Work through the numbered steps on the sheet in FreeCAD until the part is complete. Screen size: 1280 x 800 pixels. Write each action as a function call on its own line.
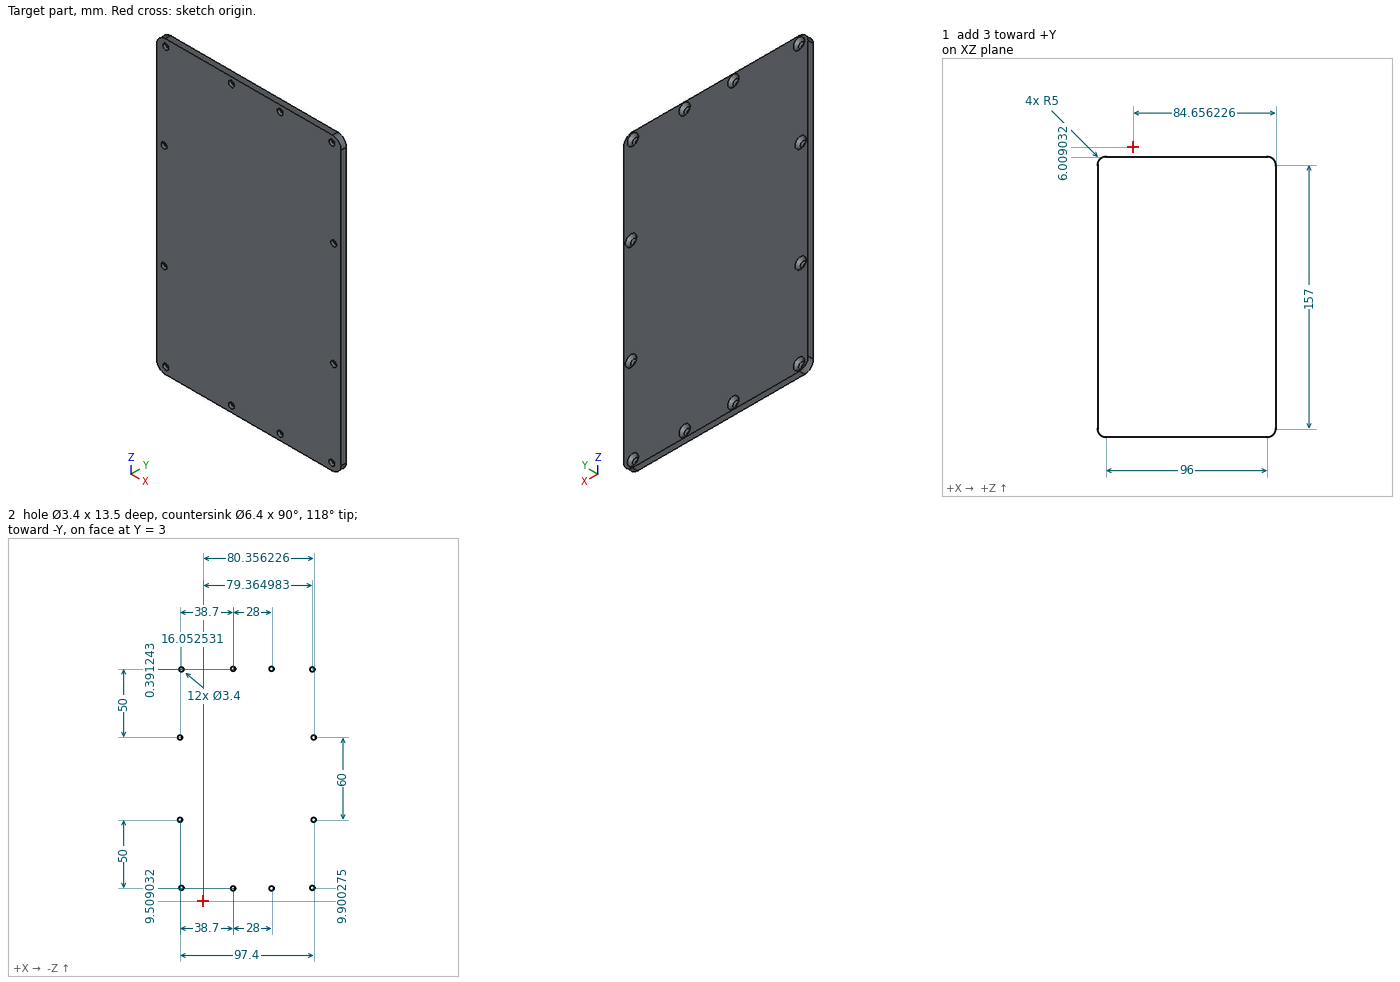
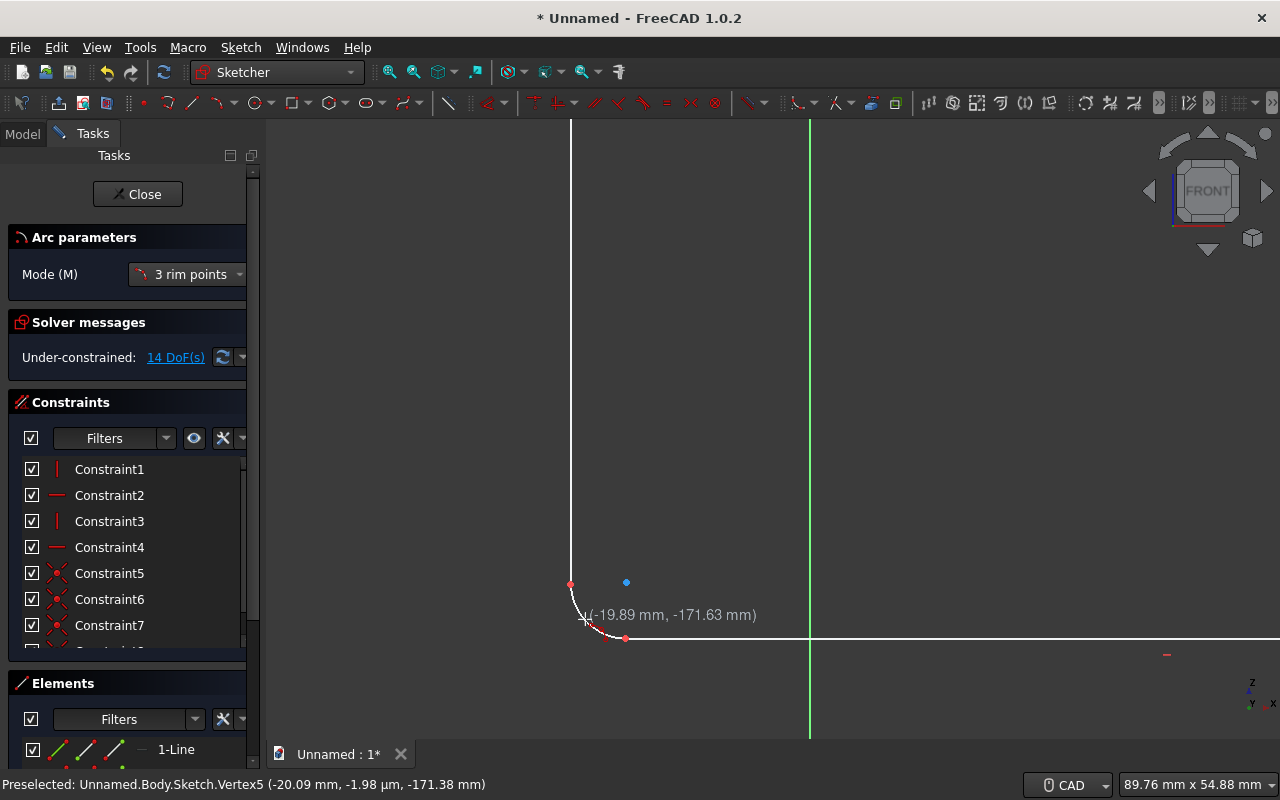
scroll(587, 624, down, 8)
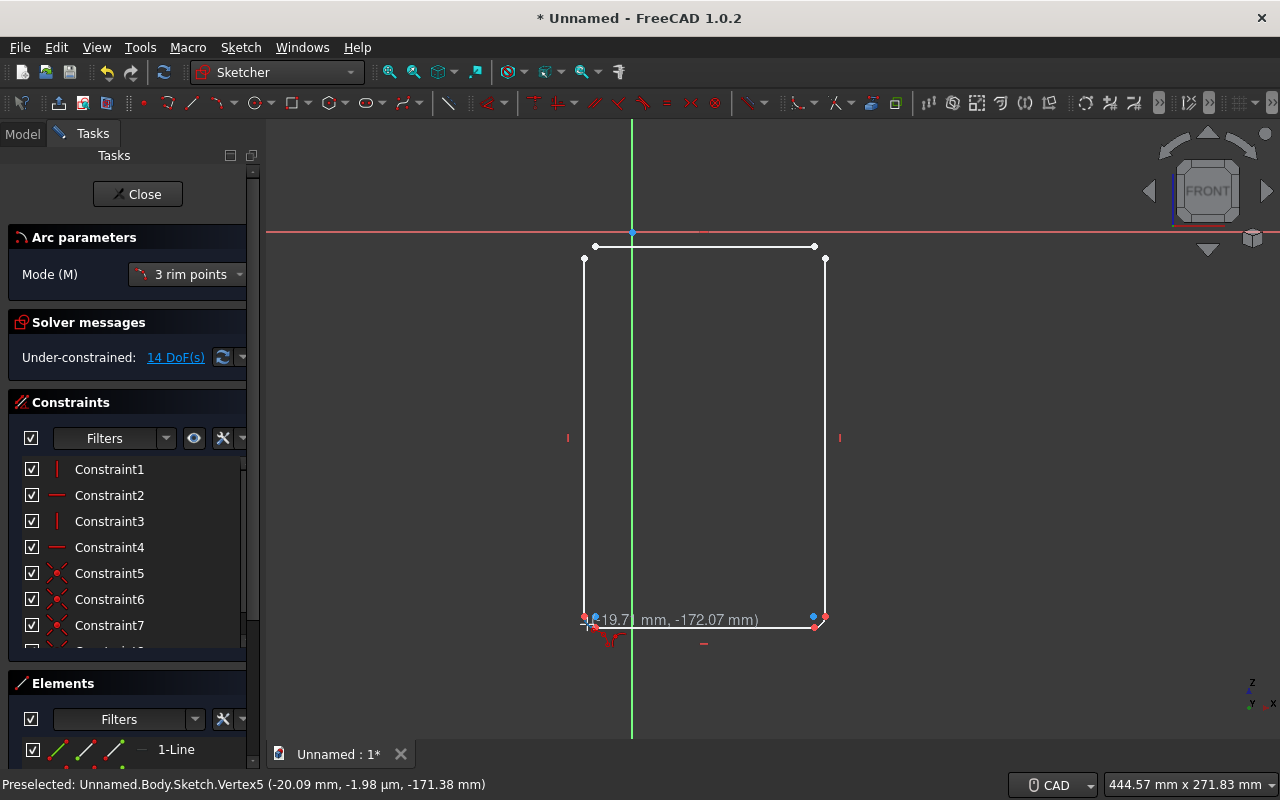
click(584, 259)
click(595, 247)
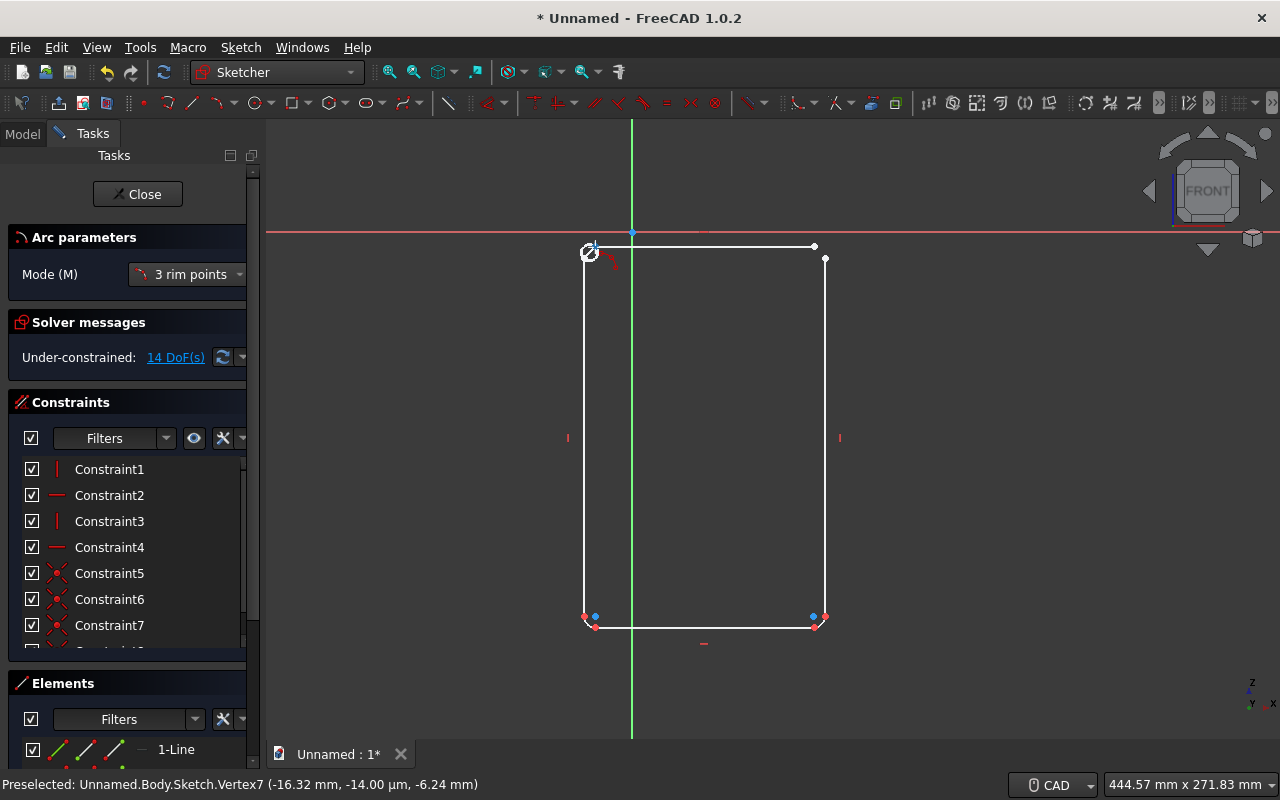
scroll(587, 249, up, 8)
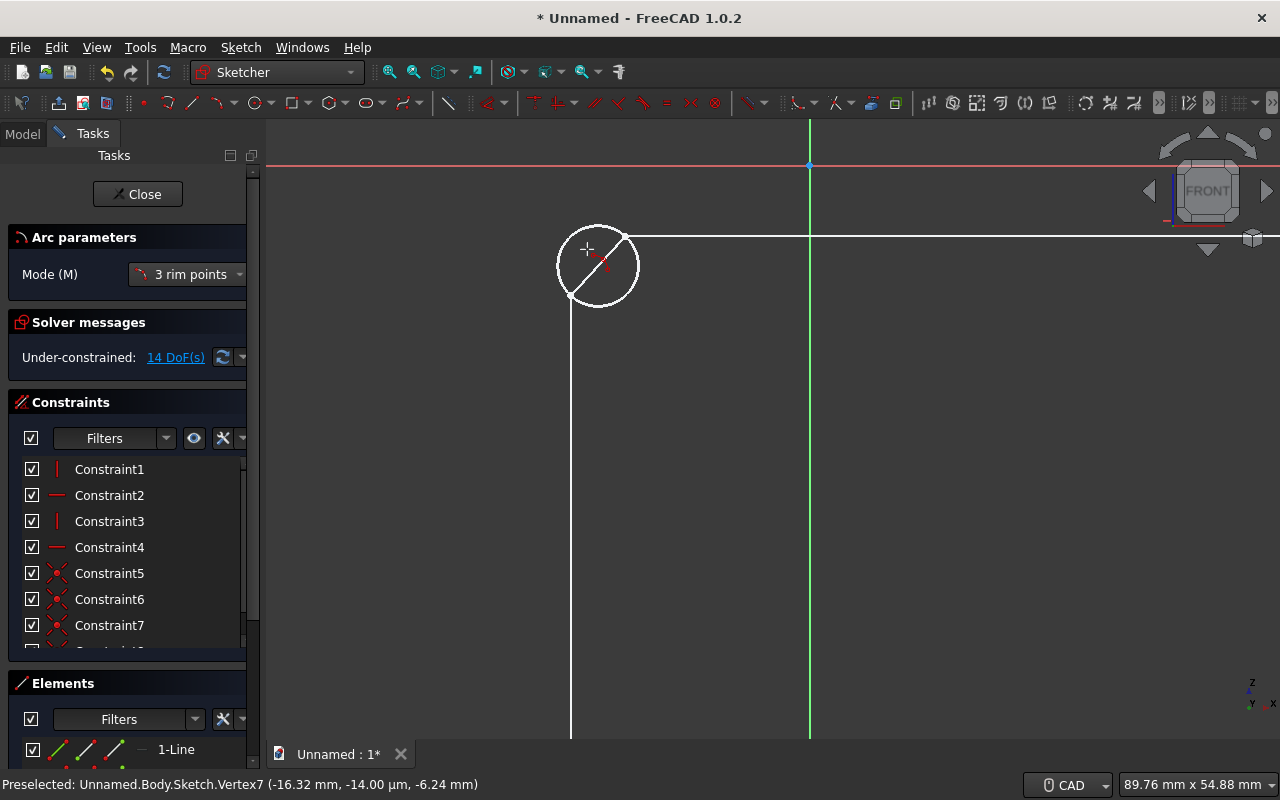
click(585, 250)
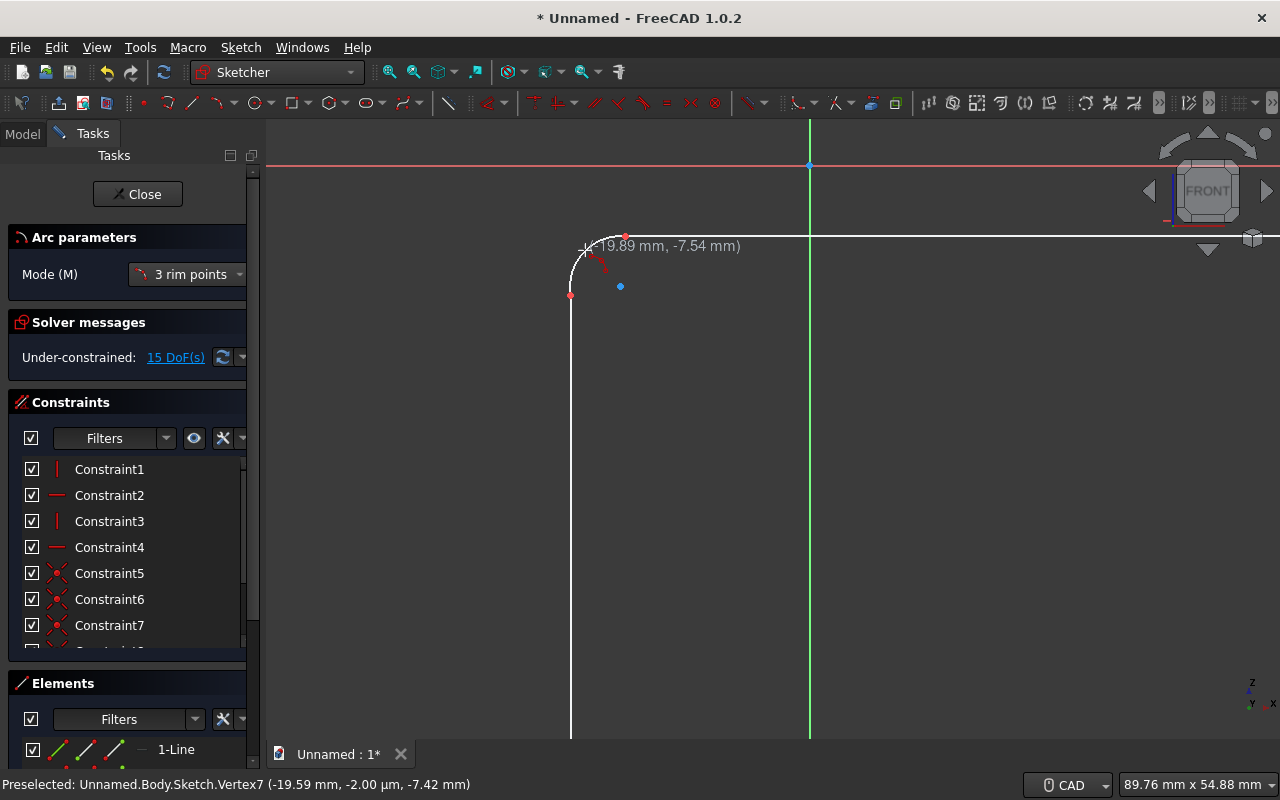
scroll(587, 248, down, 8)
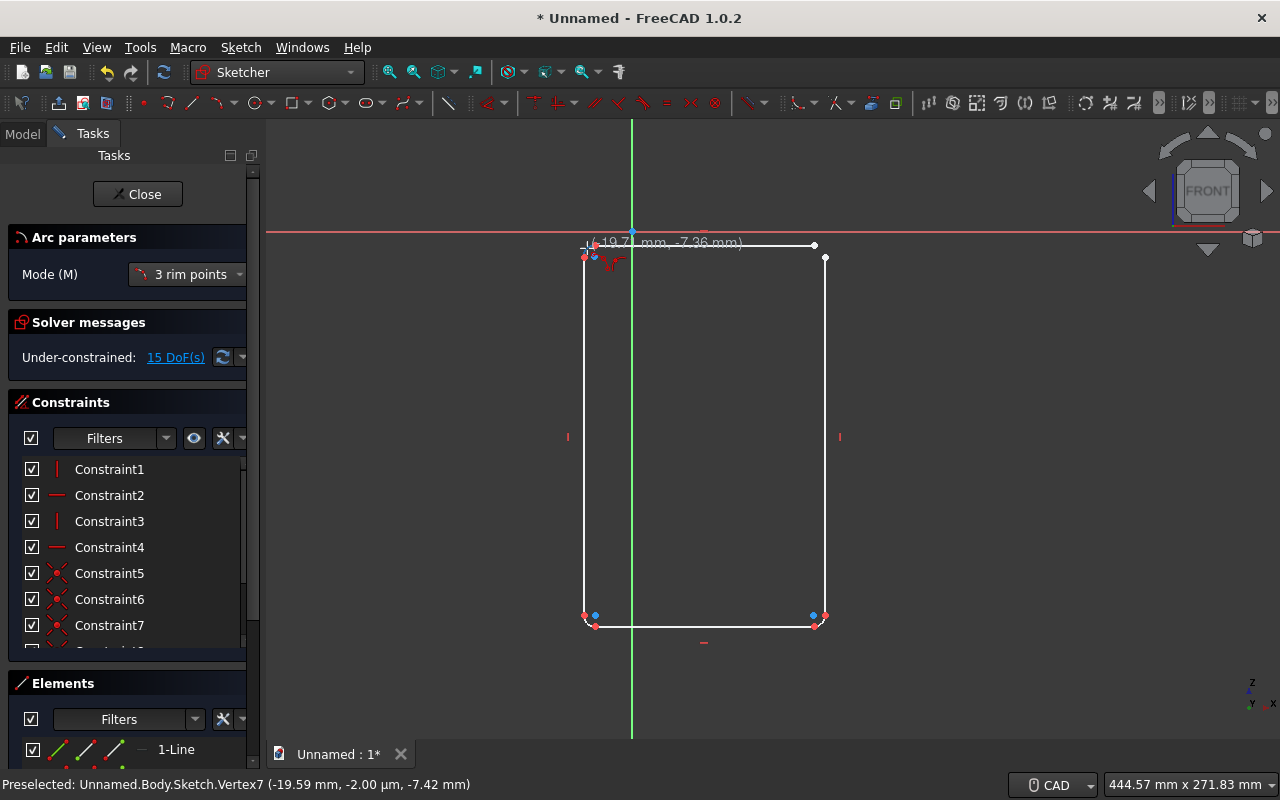
click(814, 246)
click(825, 258)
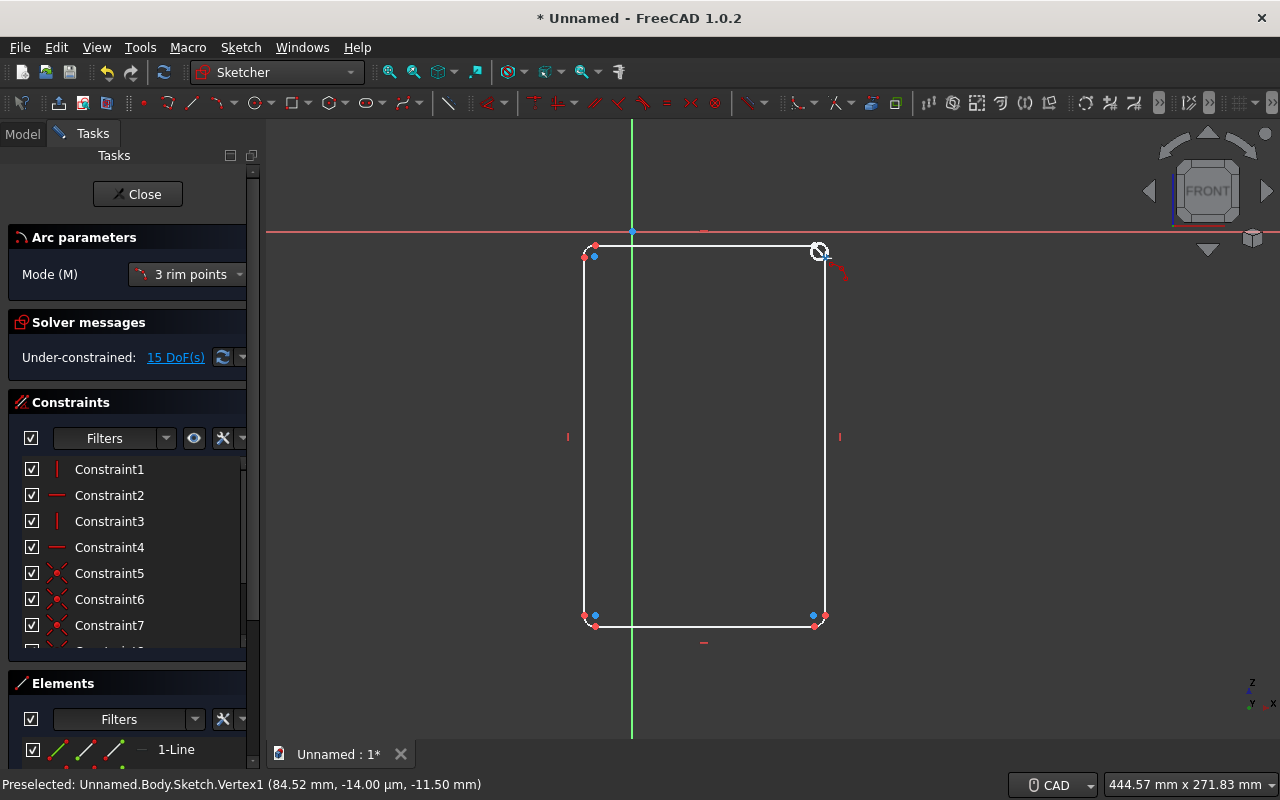
scroll(822, 249, up, 8)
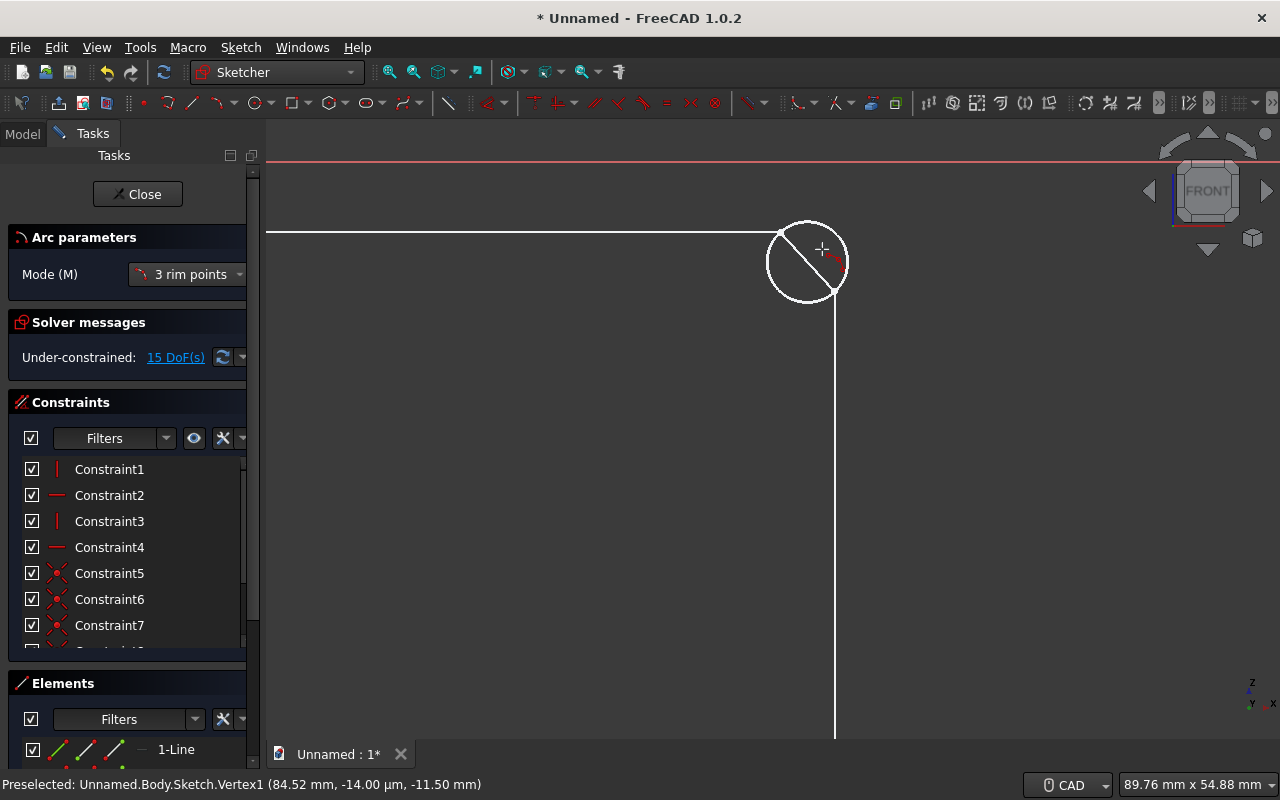
click(820, 246)
key(Escape)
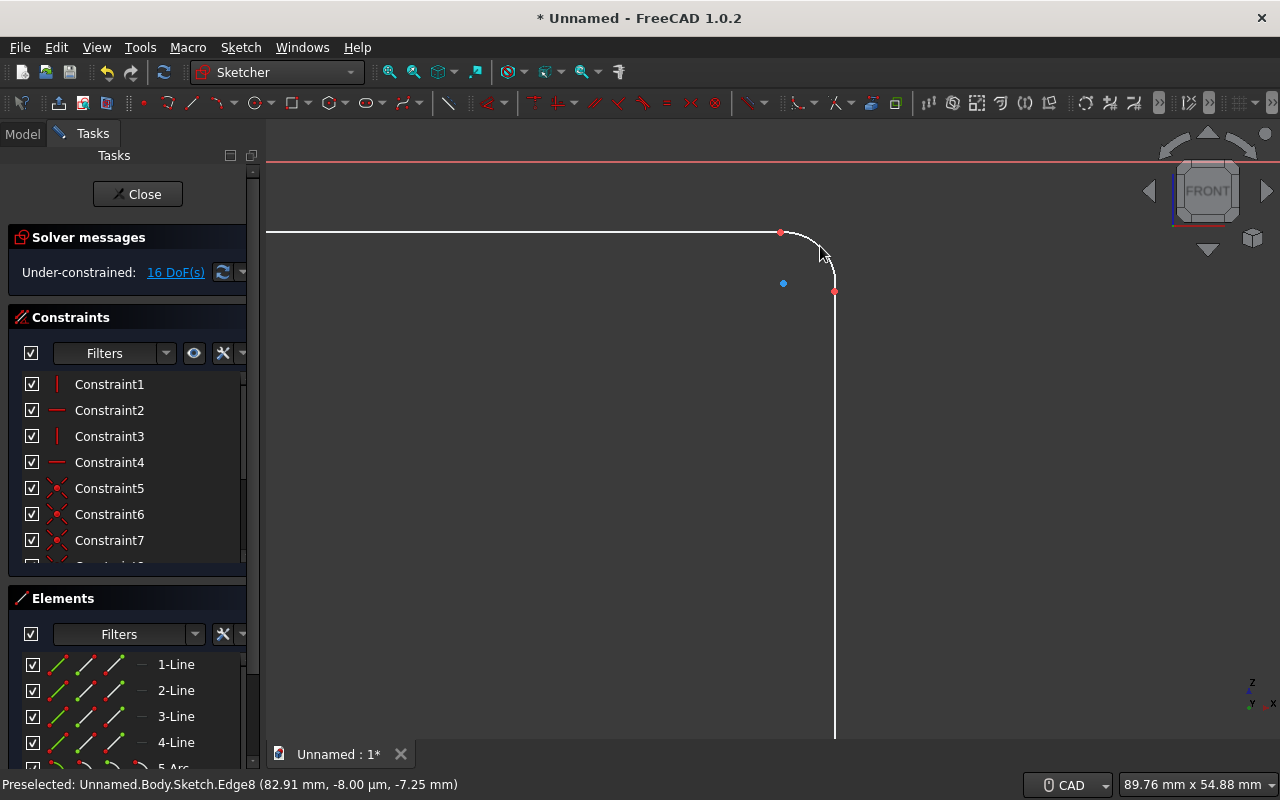
scroll(823, 249, down, 8)